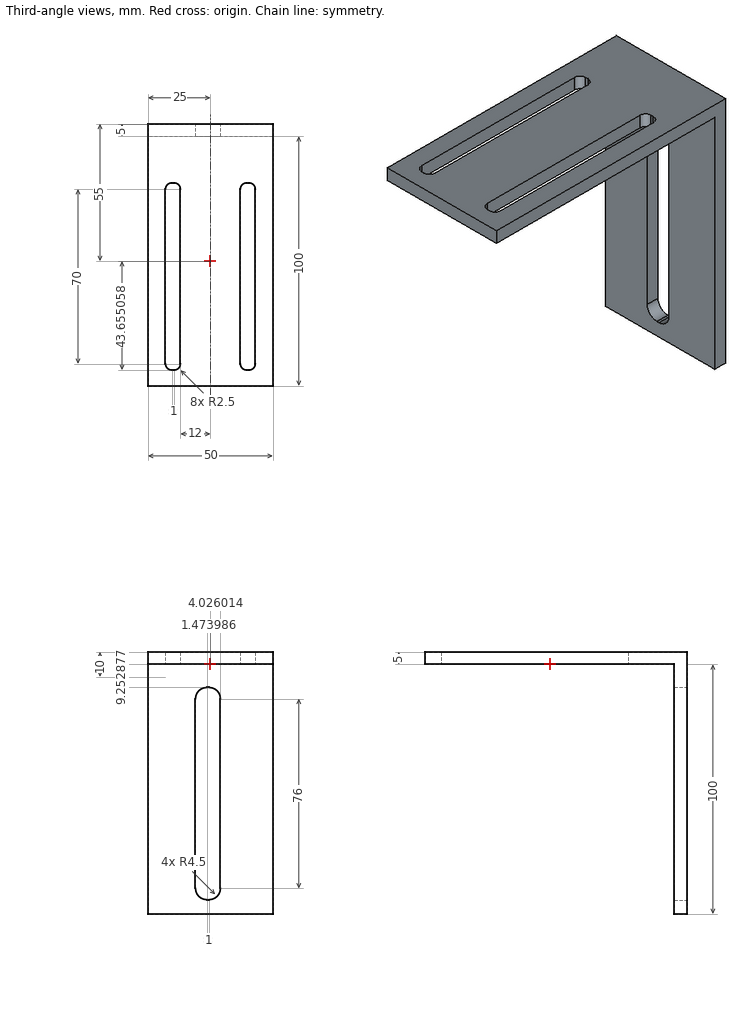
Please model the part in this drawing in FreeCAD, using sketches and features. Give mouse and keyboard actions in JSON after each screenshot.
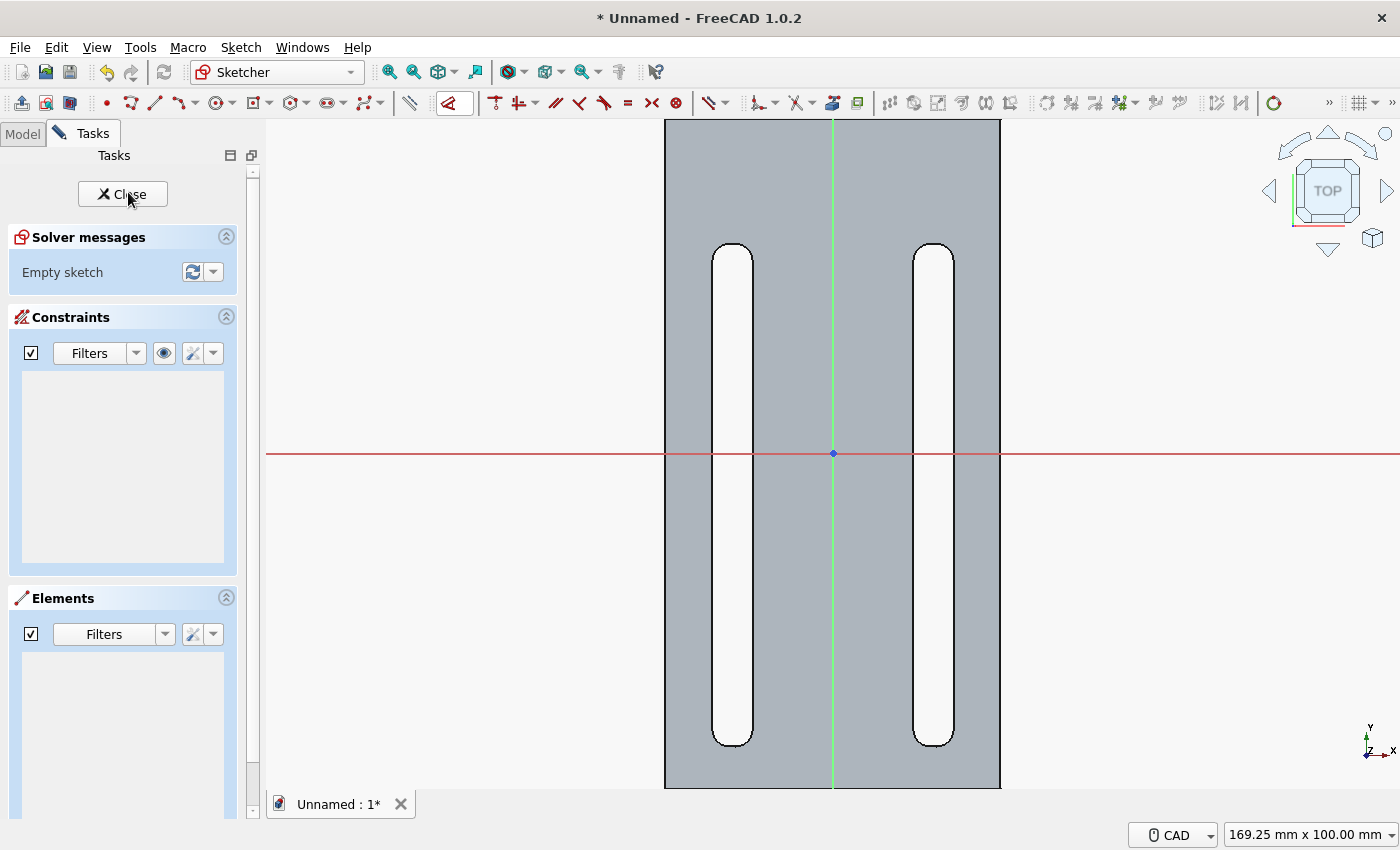
{"action": "scroll", "coordinate": [455, 761], "scroll_direction": "down", "scroll_amount": 1}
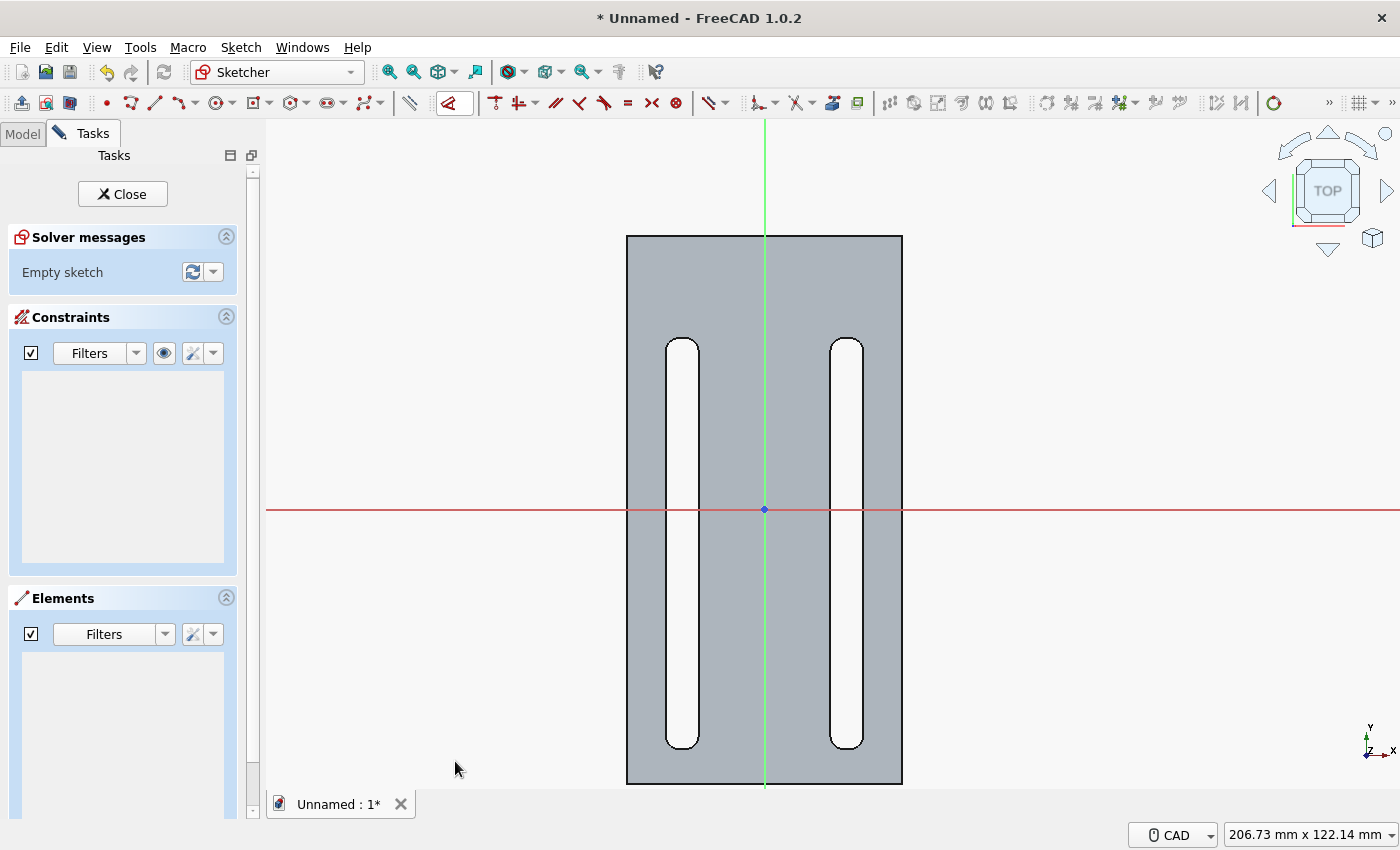
{"action": "scroll", "coordinate": [765, 166], "scroll_direction": "up", "scroll_amount": 2}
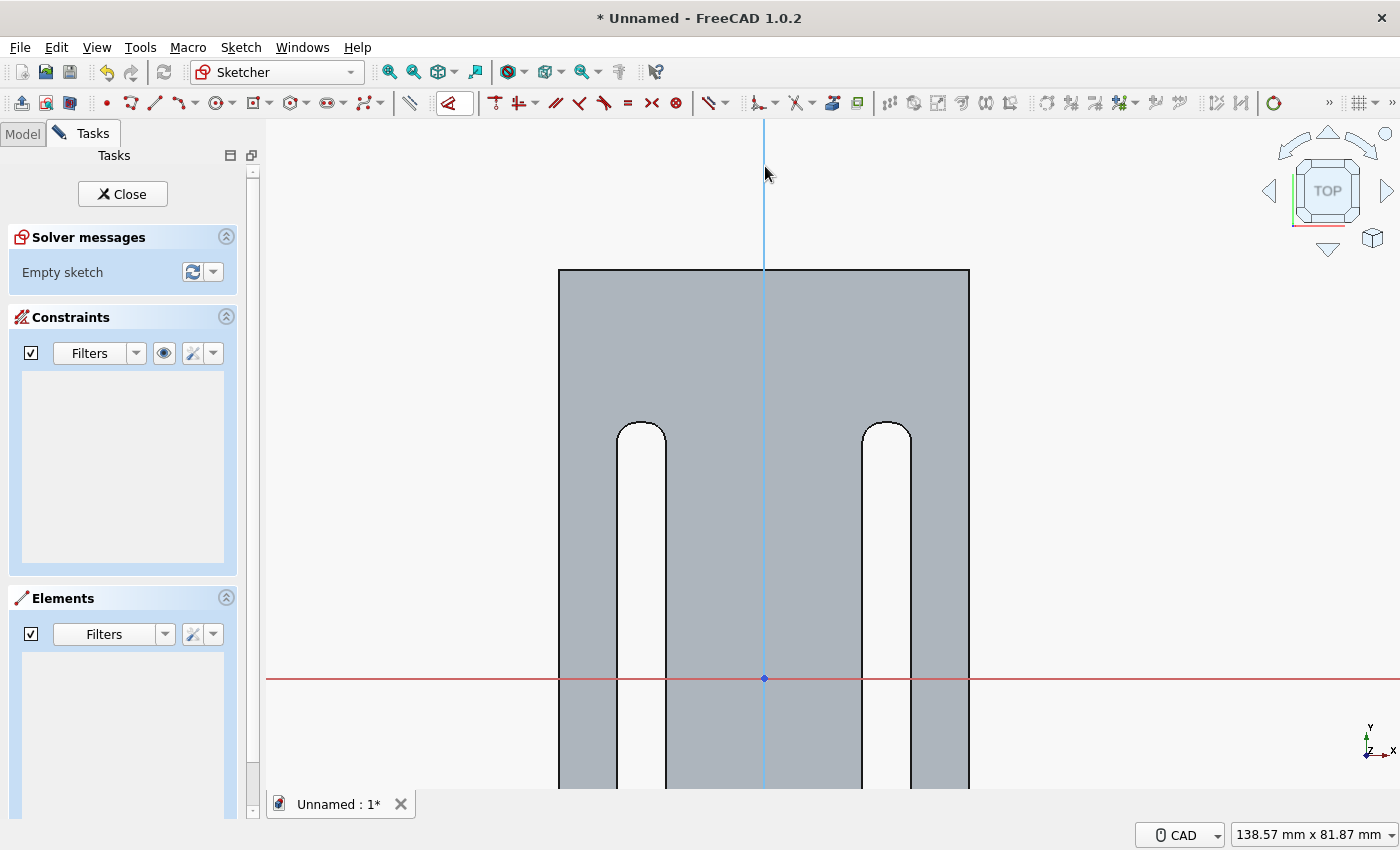
{"action": "key", "text": "g r"}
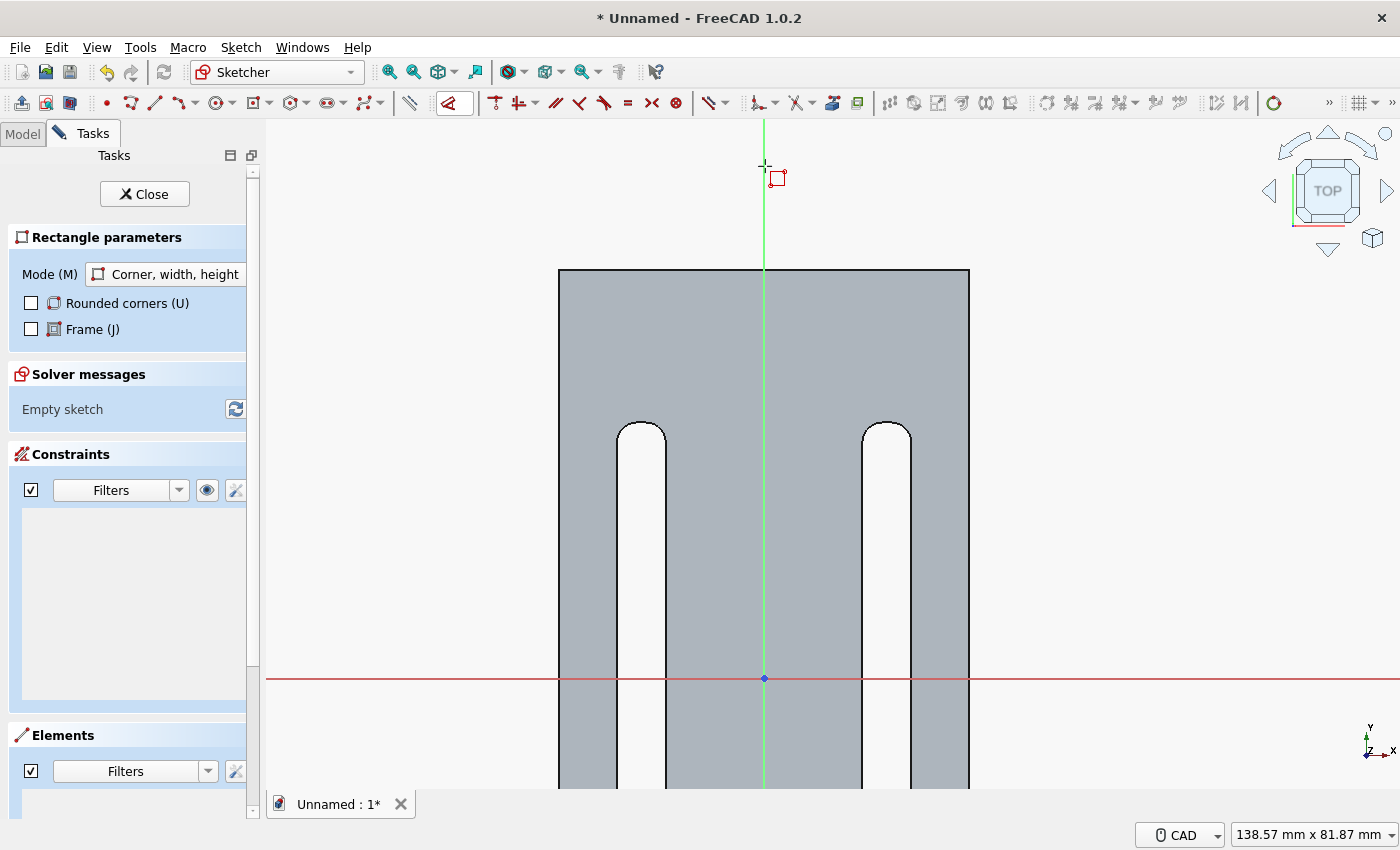
{"action": "left_click", "coordinate": [559, 229]}
{"action": "left_click", "coordinate": [969, 270]}
{"action": "key", "text": "Escape"}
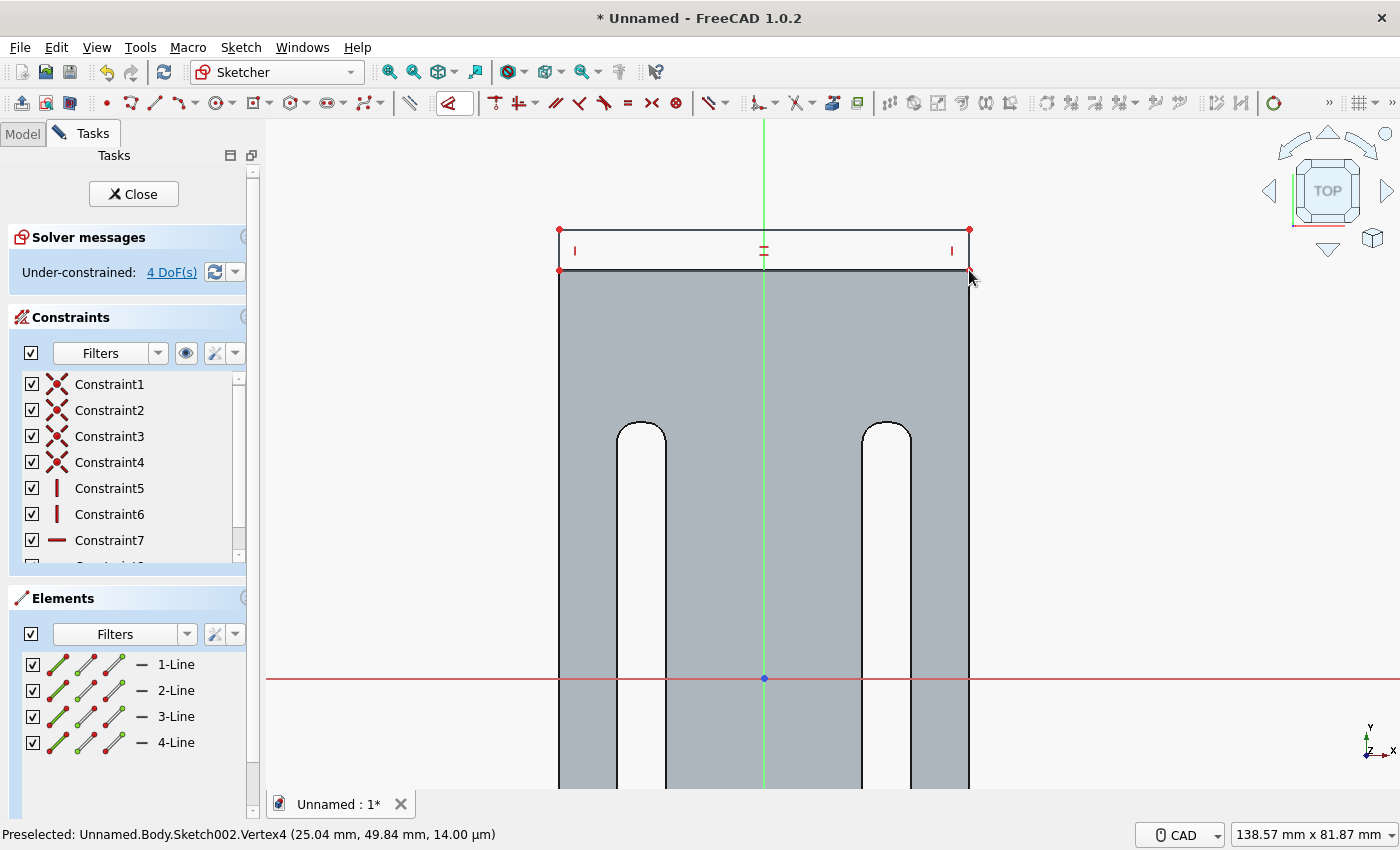
{"action": "left_click", "coordinate": [559, 242]}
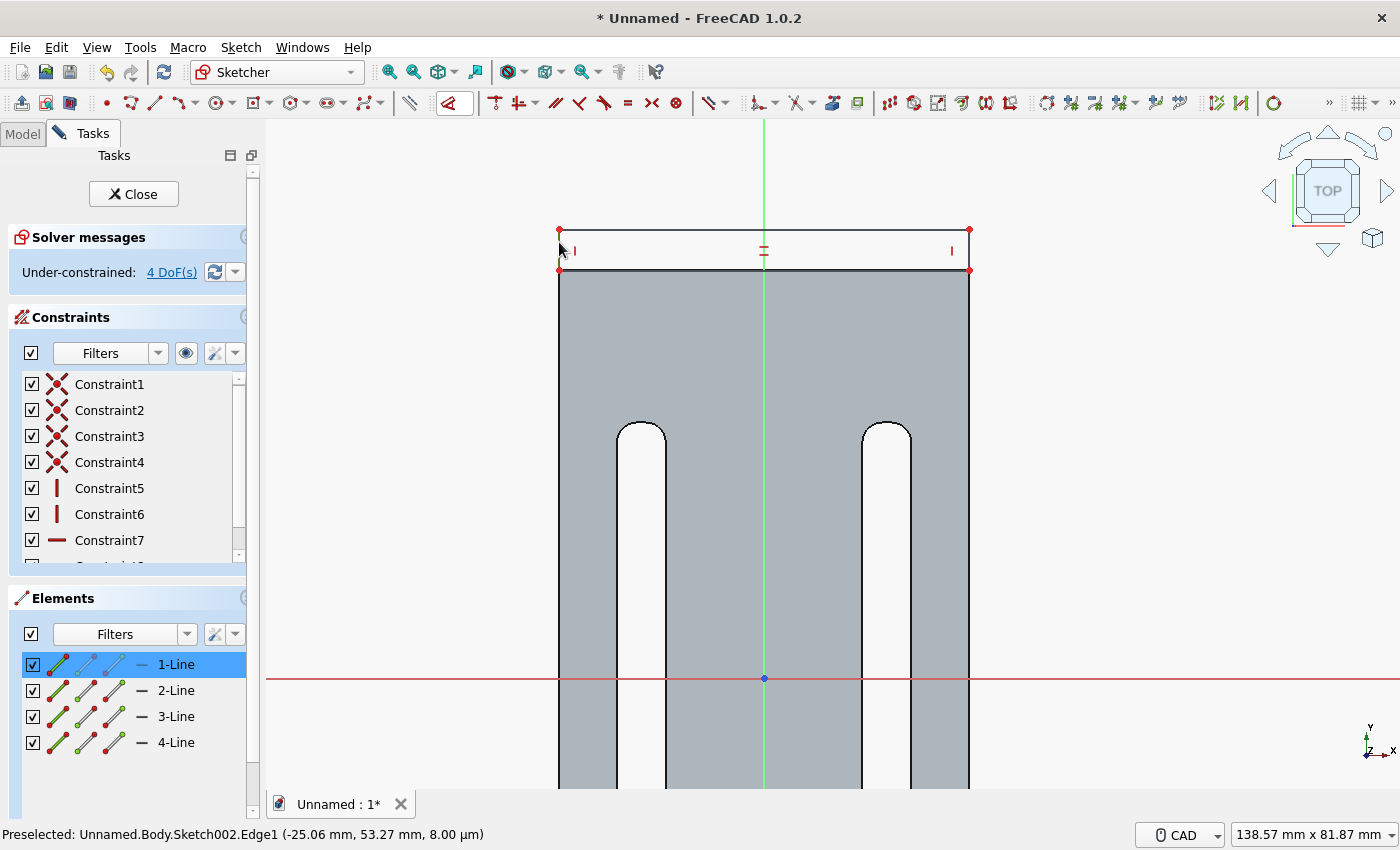
{"action": "key", "text": "i"}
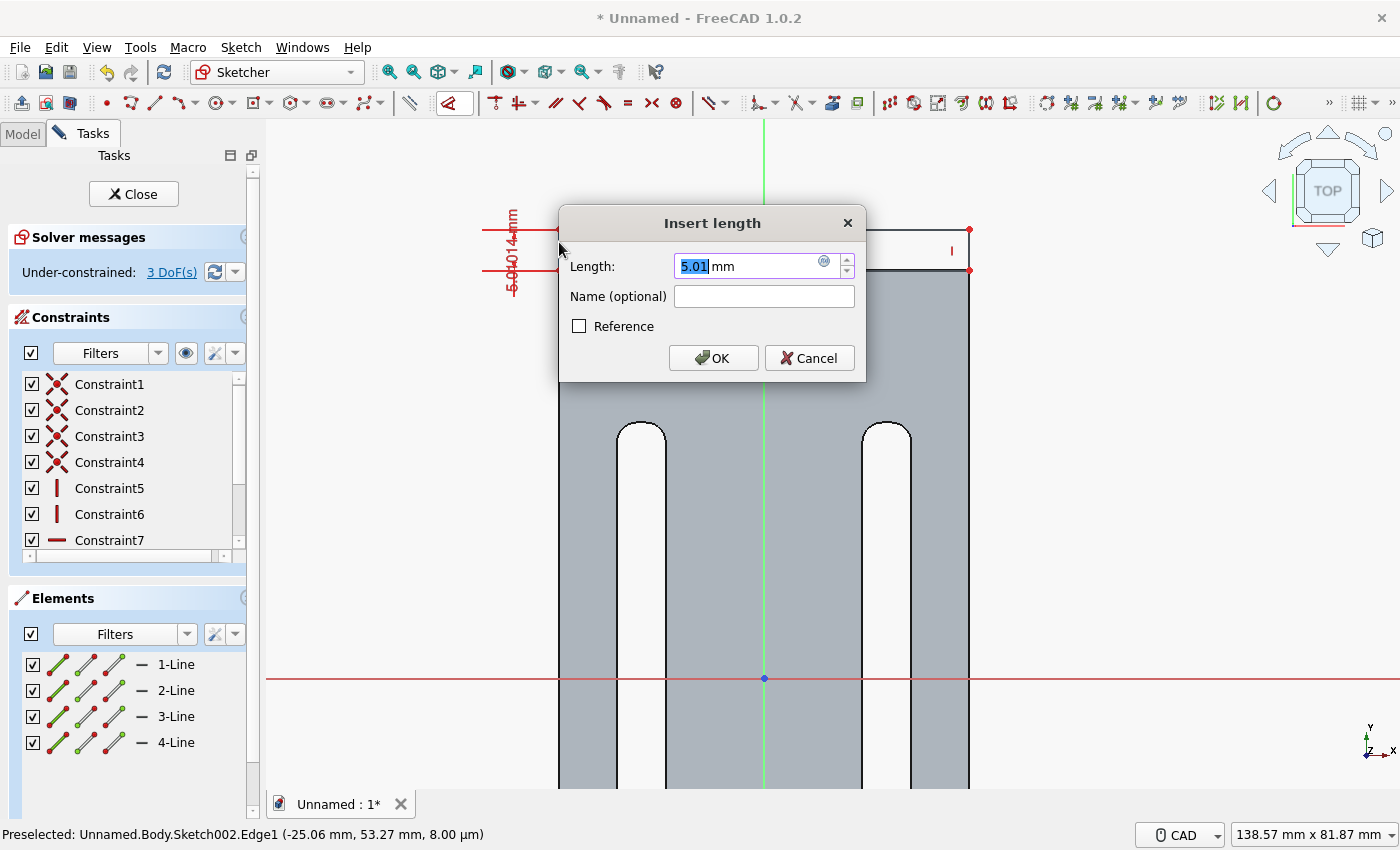
{"action": "type", "text": "5"}
{"action": "key", "text": "Return"}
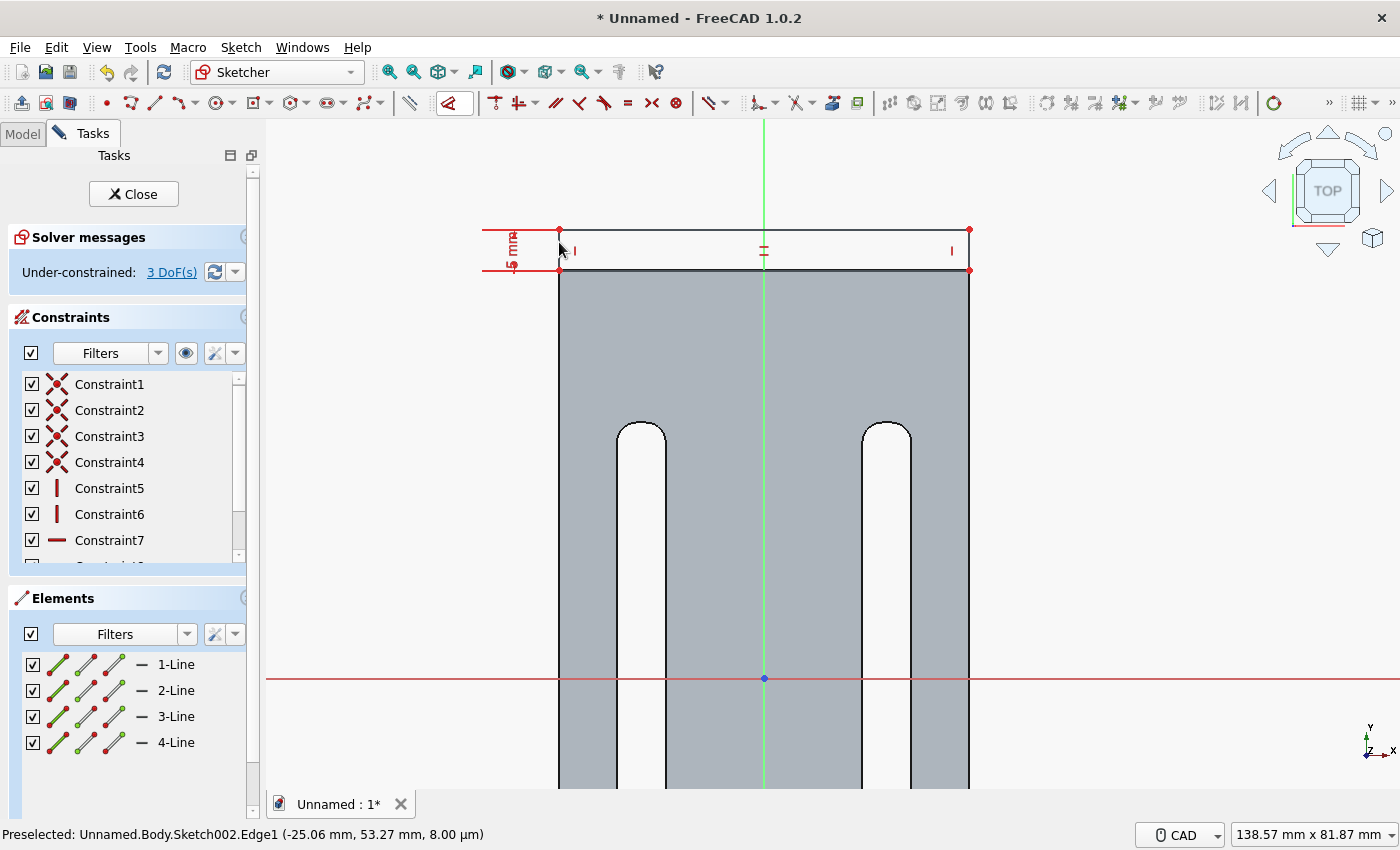
{"action": "left_click", "coordinate": [682, 271]}